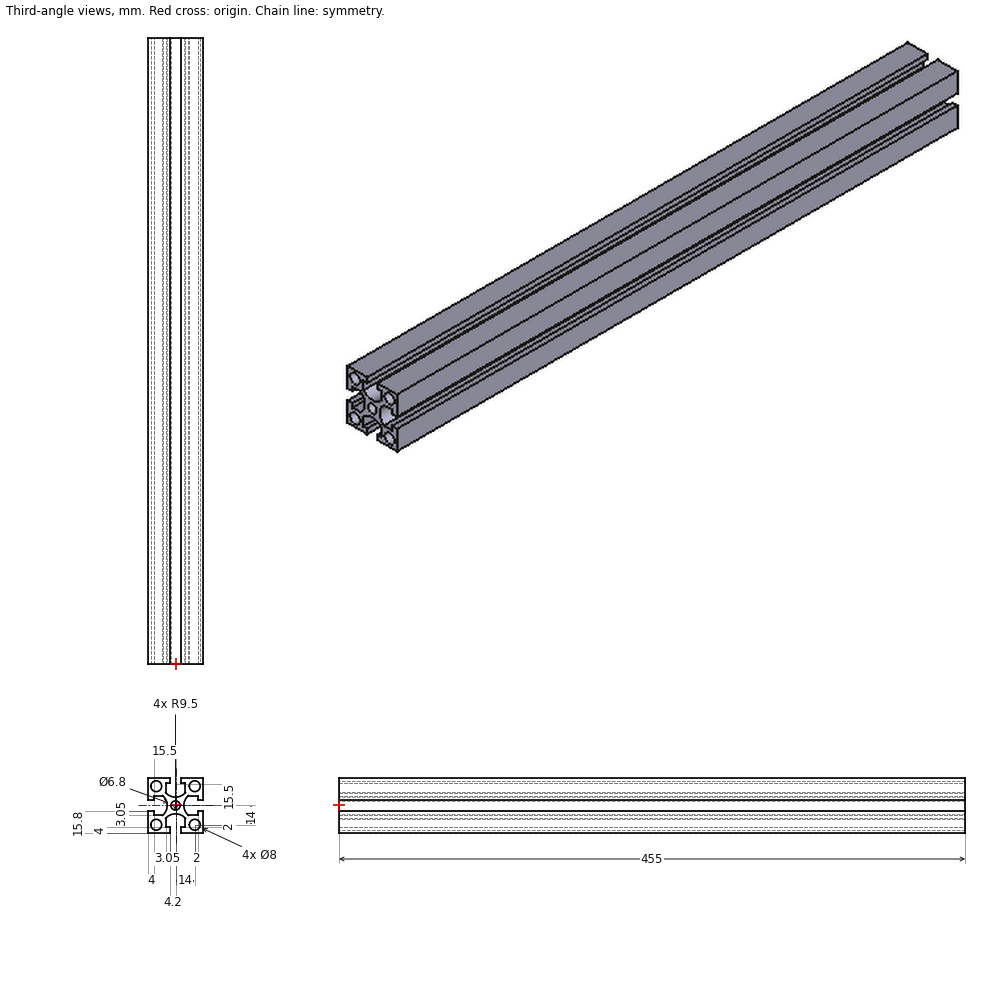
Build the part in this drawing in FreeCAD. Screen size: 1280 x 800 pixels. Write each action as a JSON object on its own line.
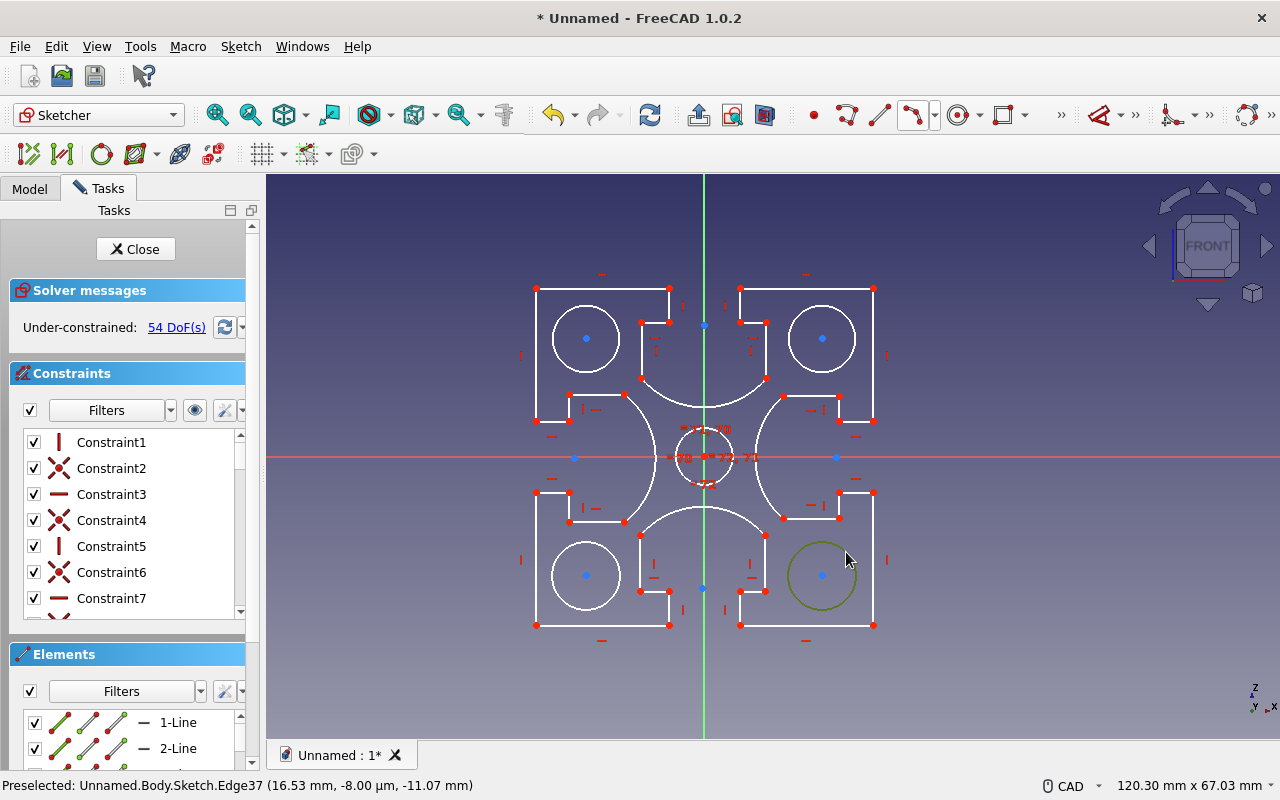
{"action": "left_click", "coordinate": [610, 552]}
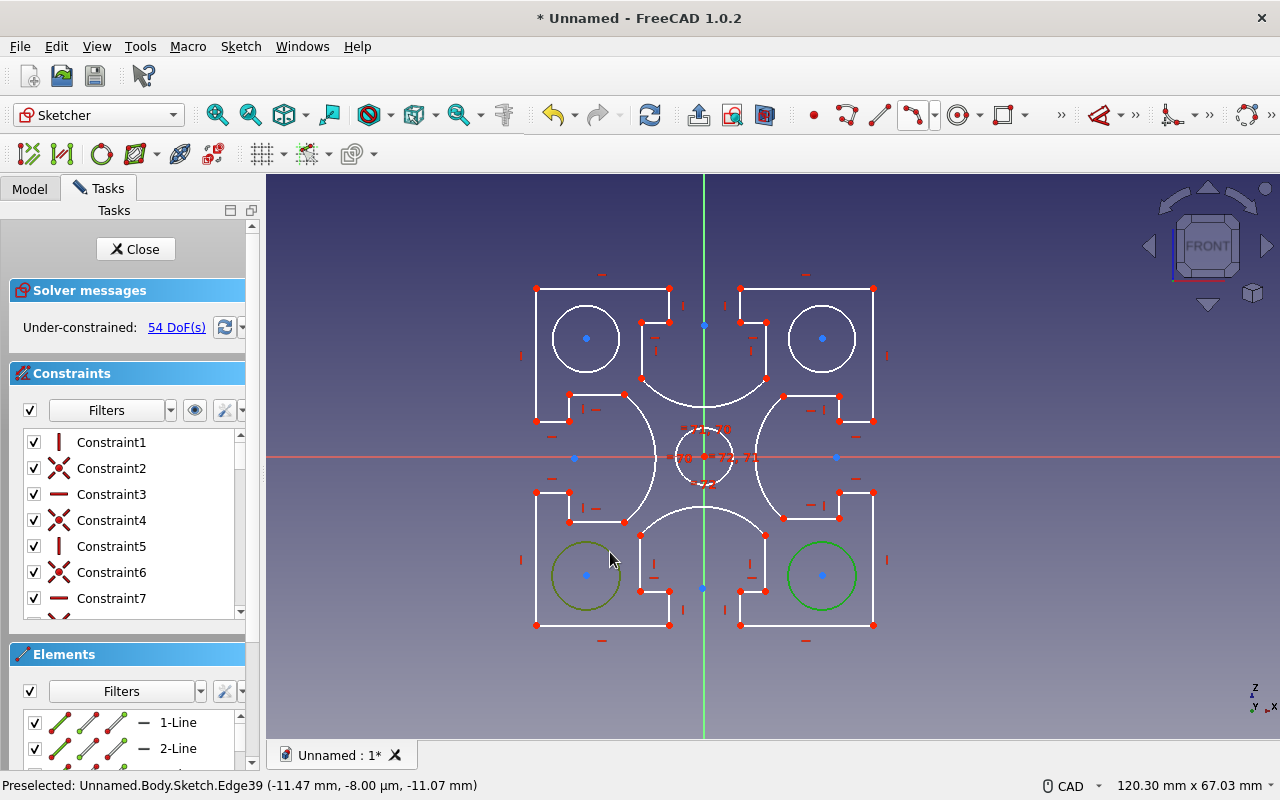
{"action": "left_click", "coordinate": [845, 315]}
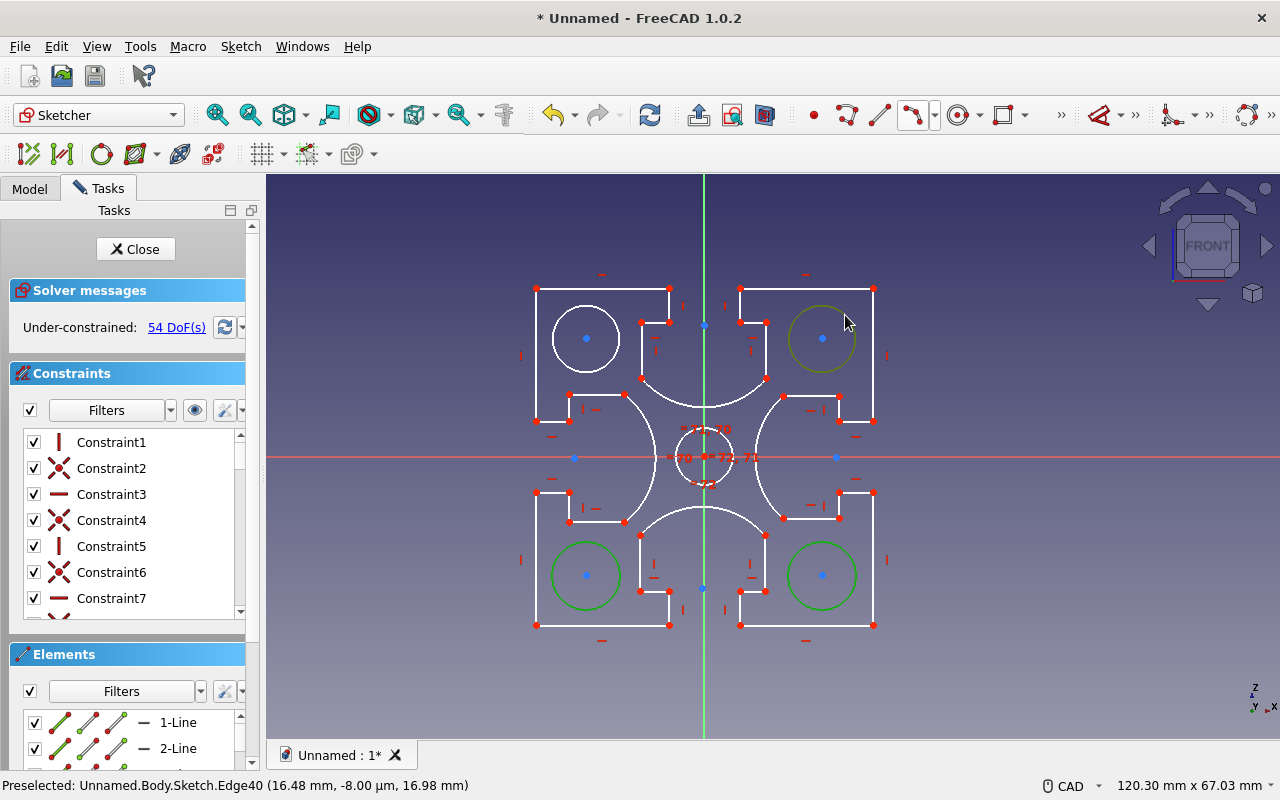
{"action": "left_click", "coordinate": [609, 315]}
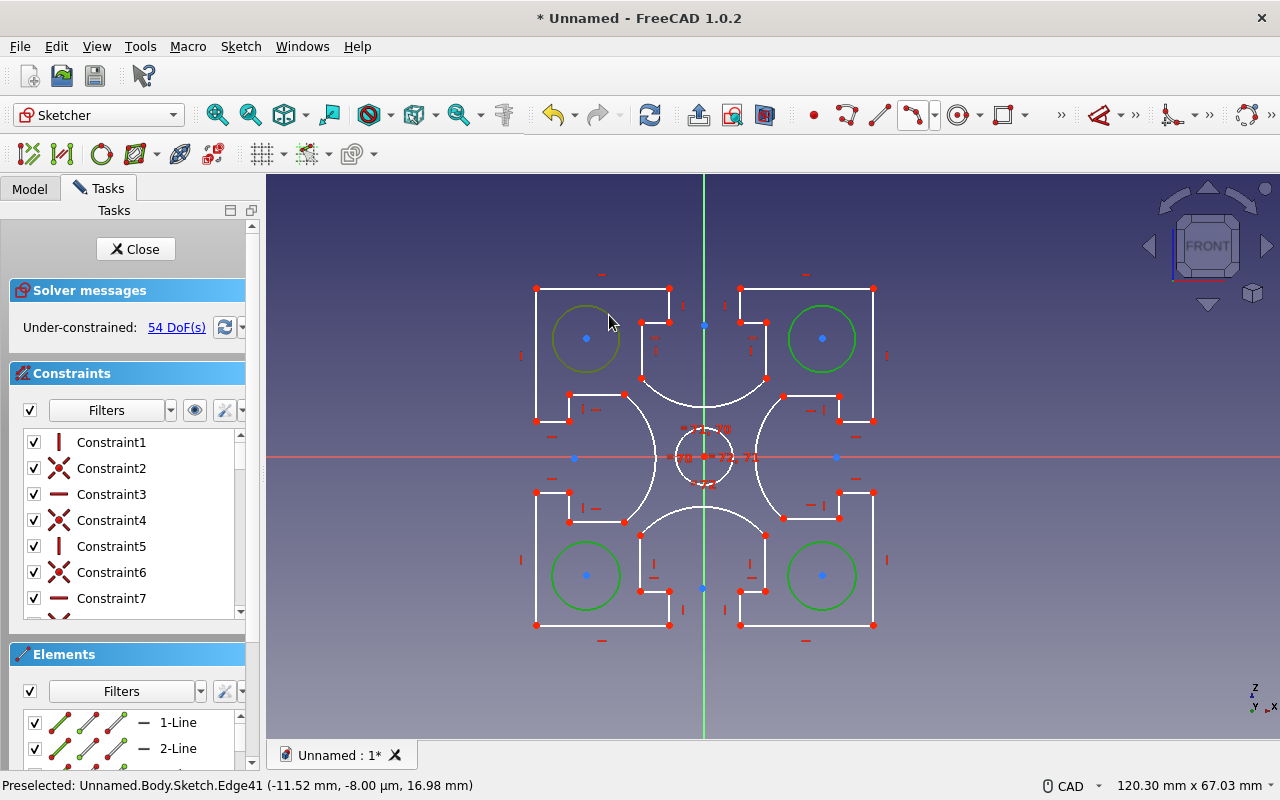
{"action": "key", "text": "e"}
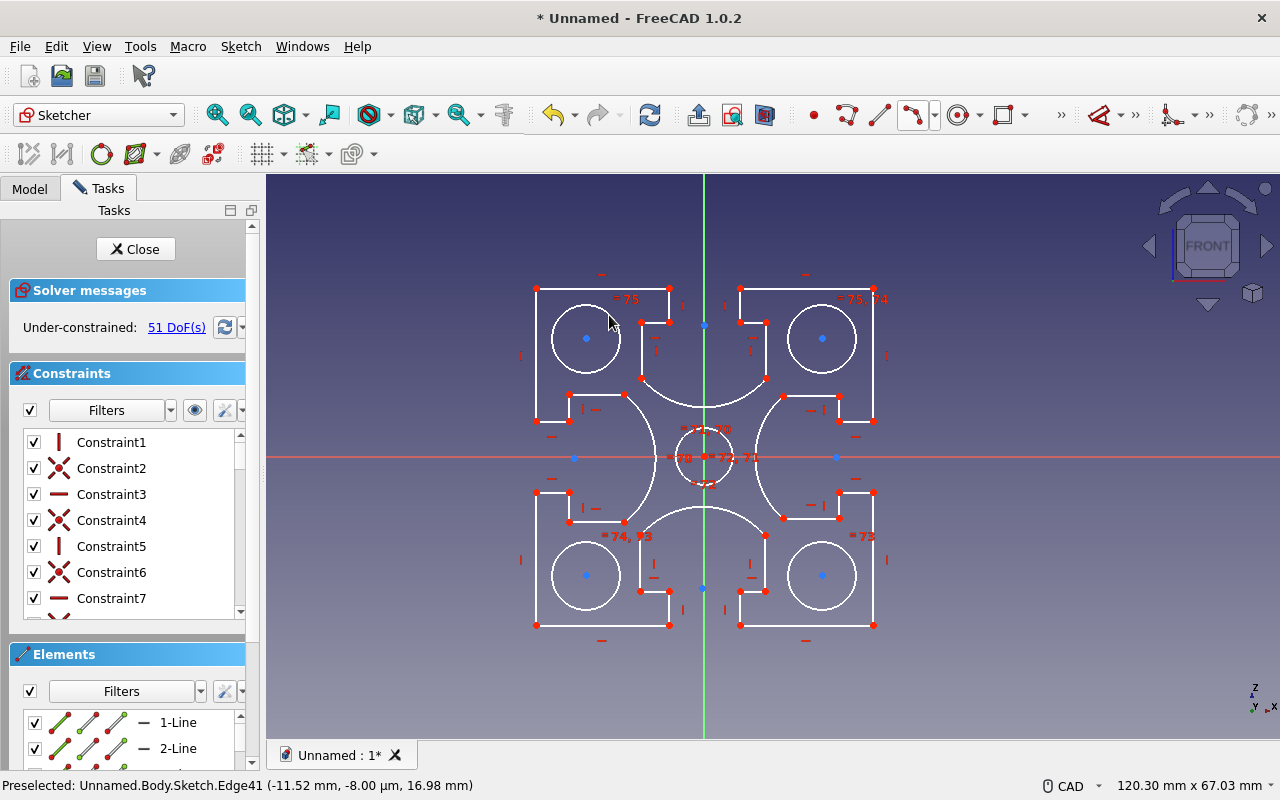
{"action": "left_click", "coordinate": [574, 459]}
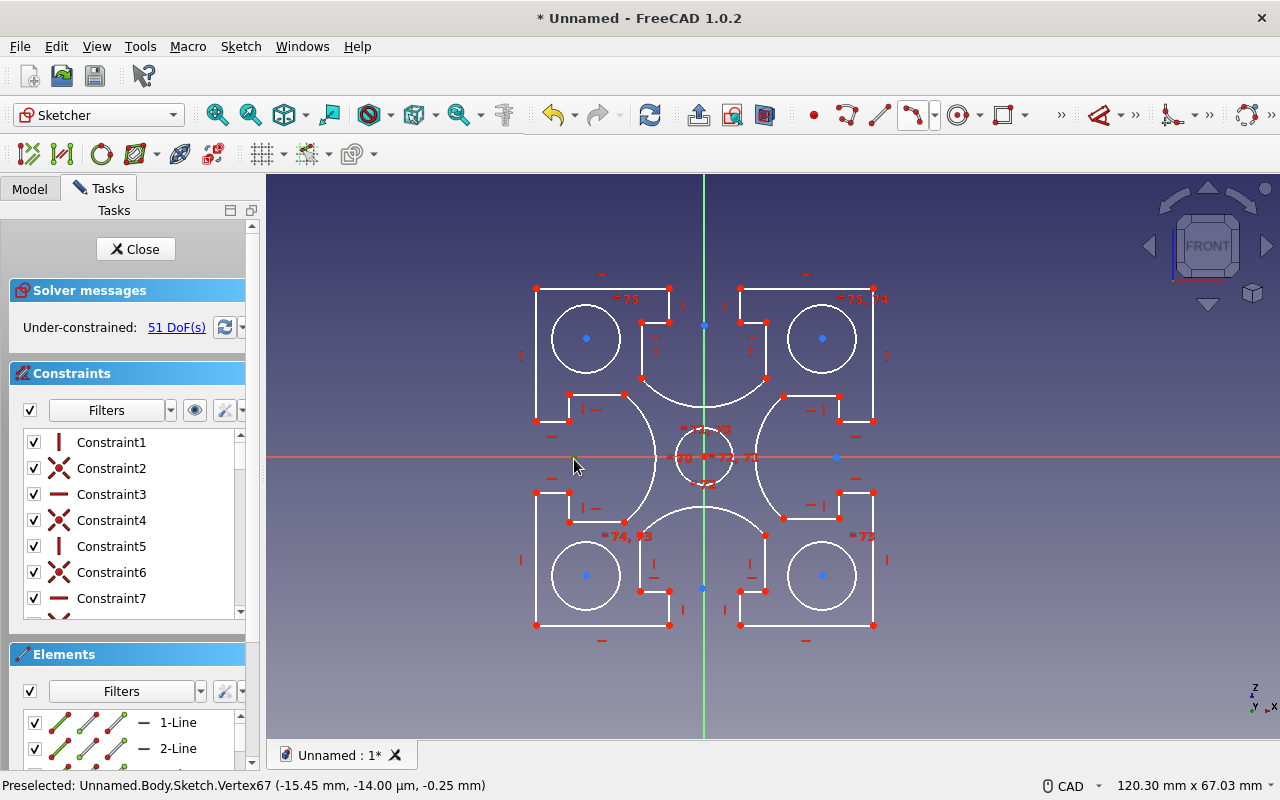
{"action": "left_click", "coordinate": [353, 456]}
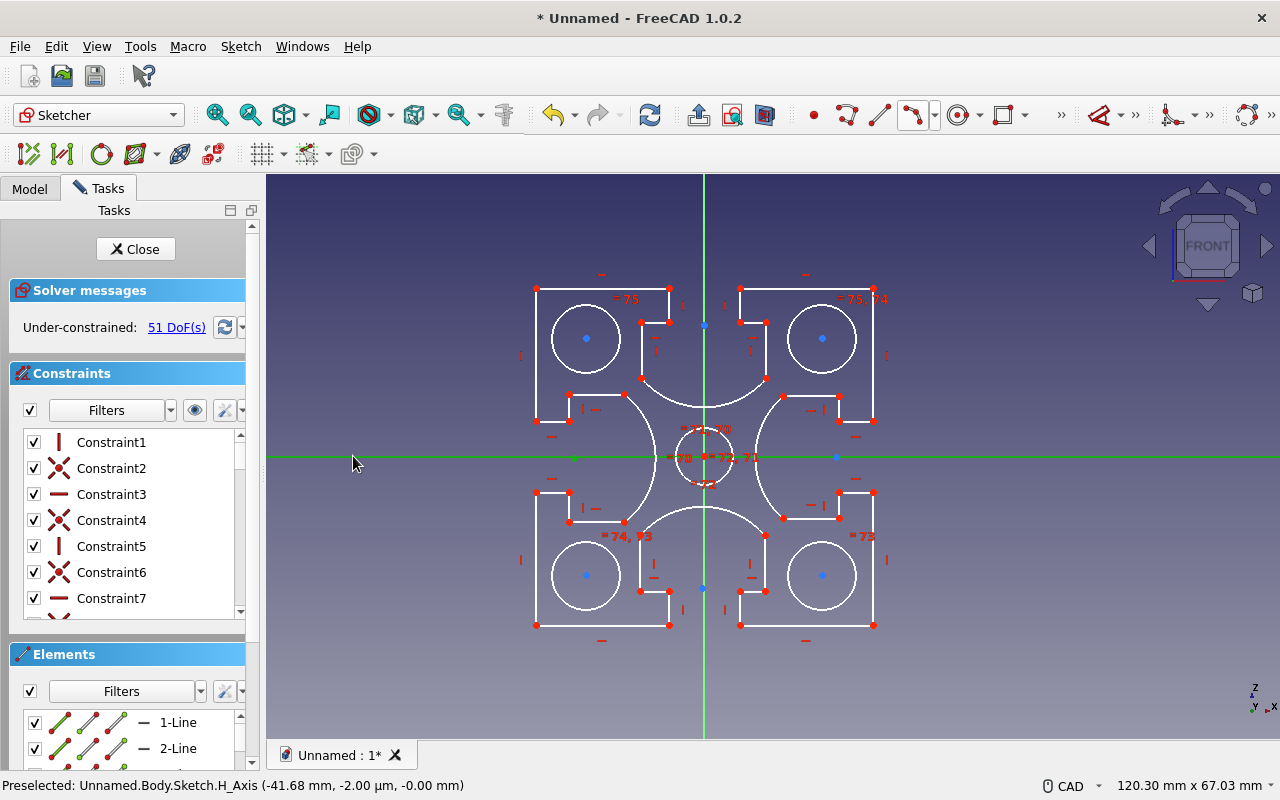
{"action": "key", "text": "c"}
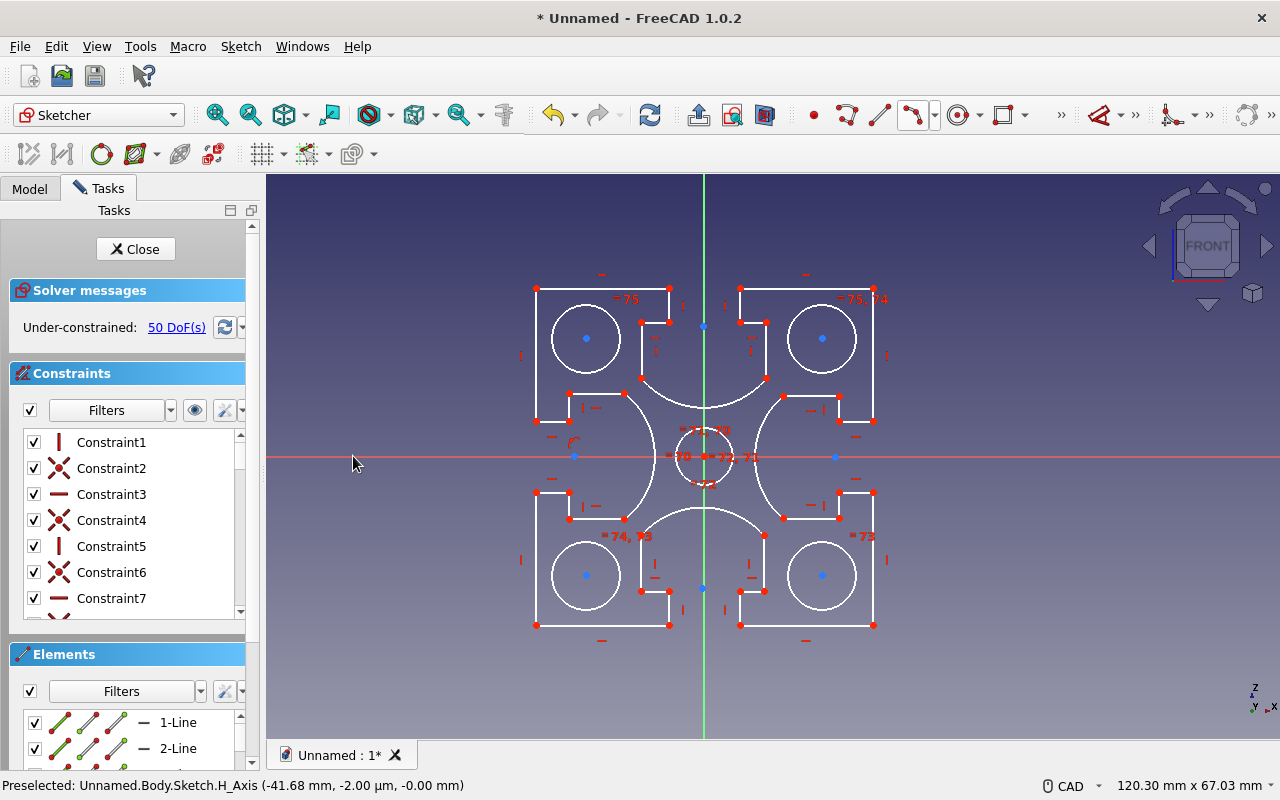
{"action": "left_click", "coordinate": [704, 327]}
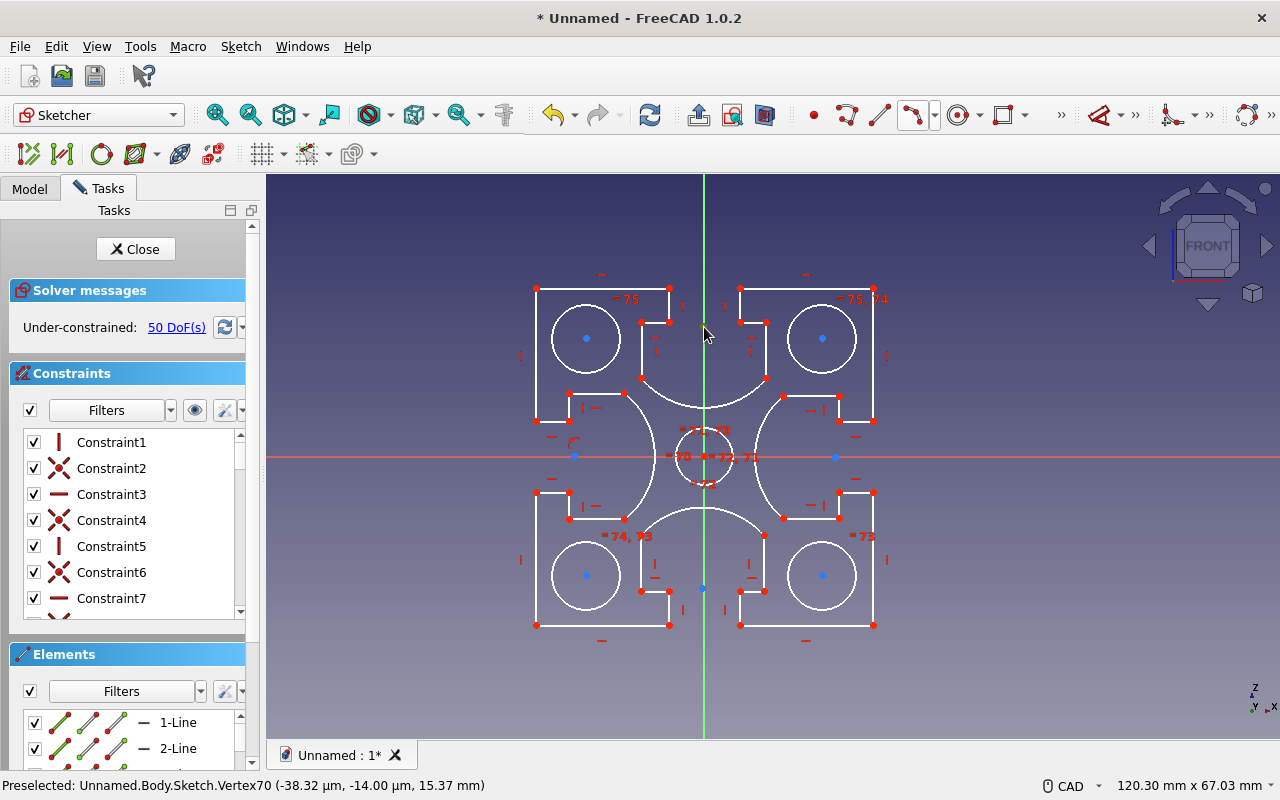
{"action": "left_click", "coordinate": [704, 675]}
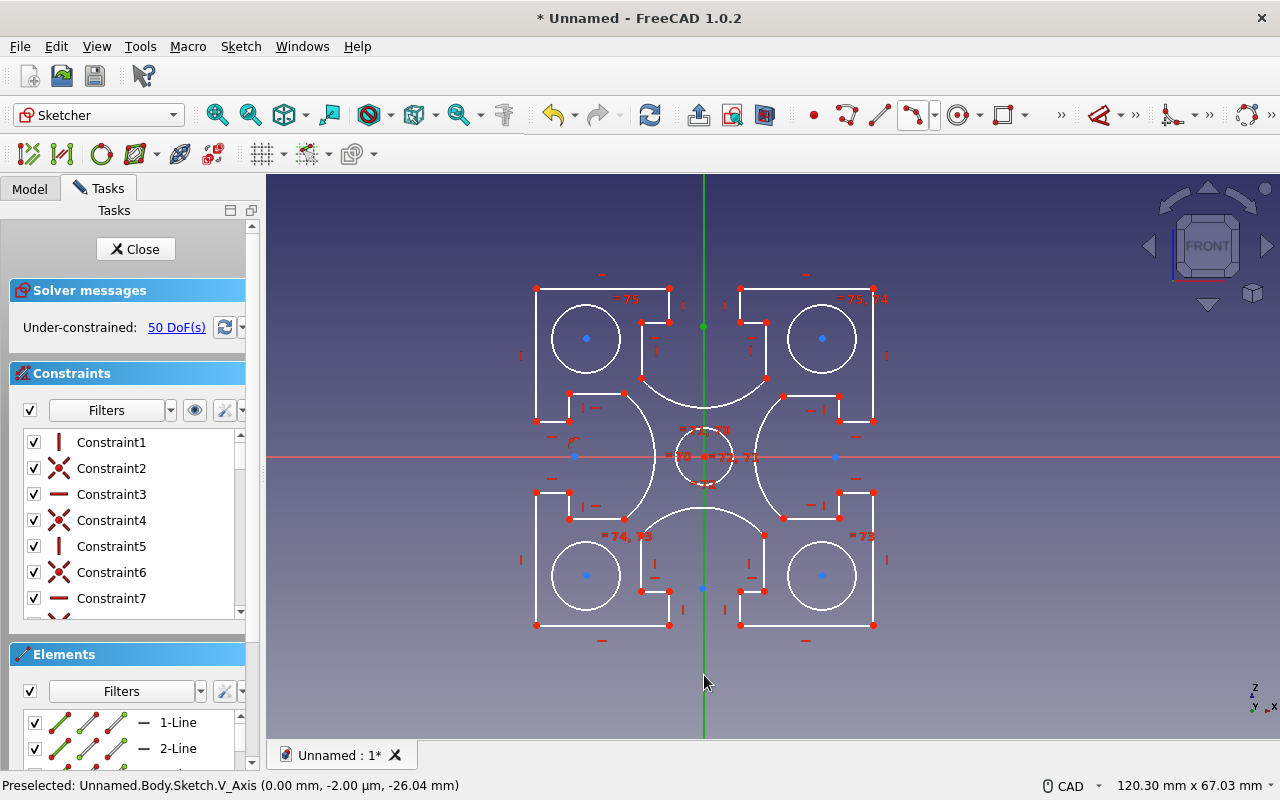
{"action": "key", "text": "c"}